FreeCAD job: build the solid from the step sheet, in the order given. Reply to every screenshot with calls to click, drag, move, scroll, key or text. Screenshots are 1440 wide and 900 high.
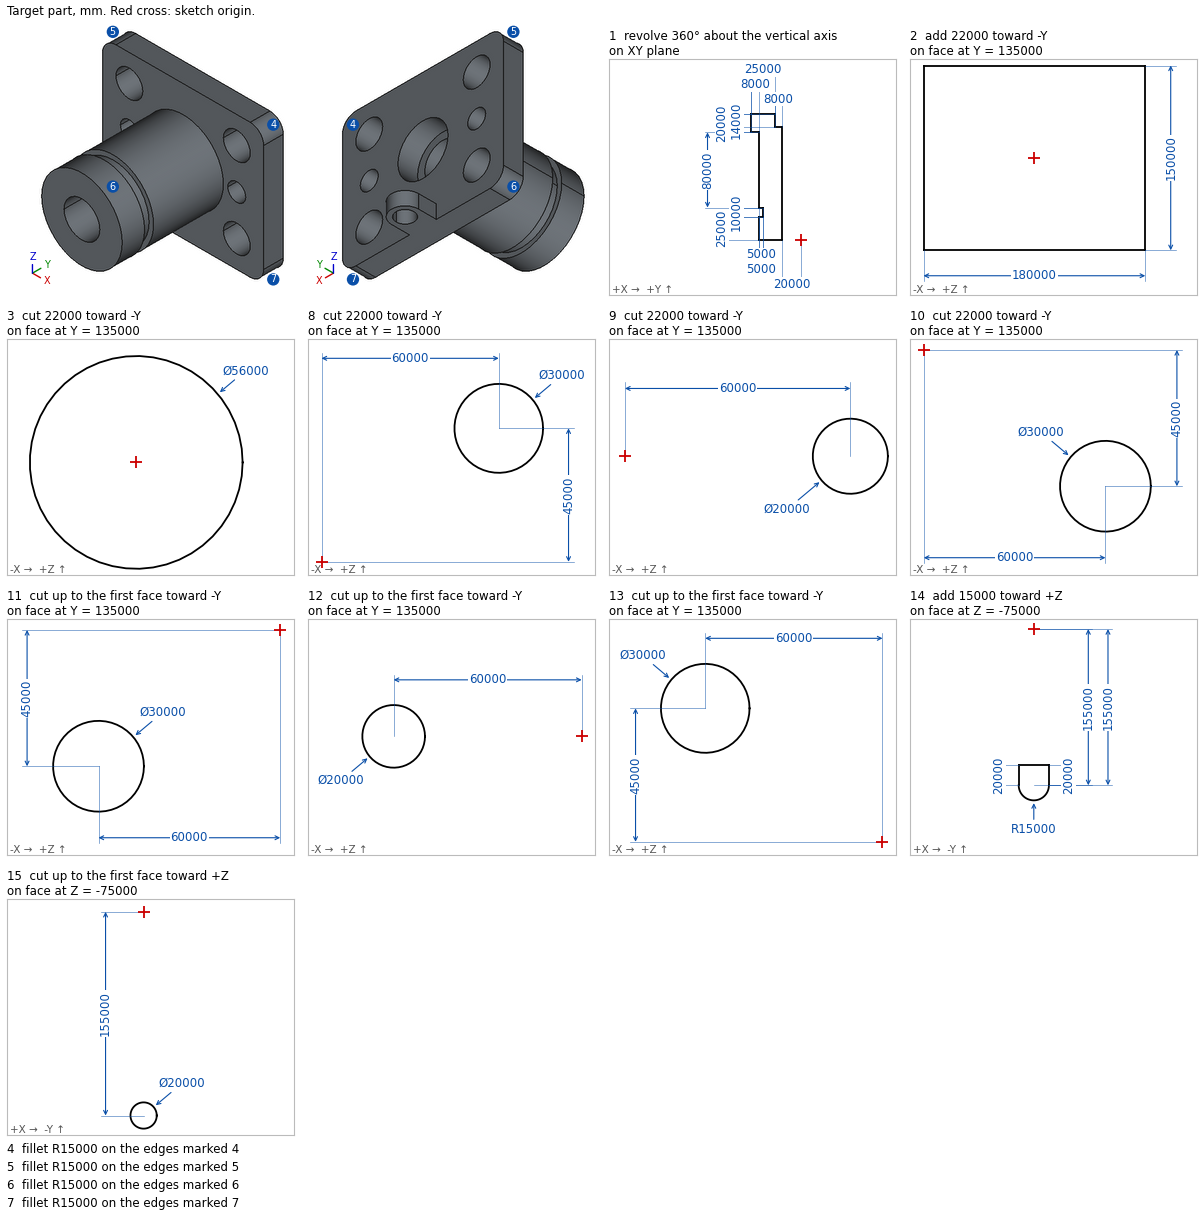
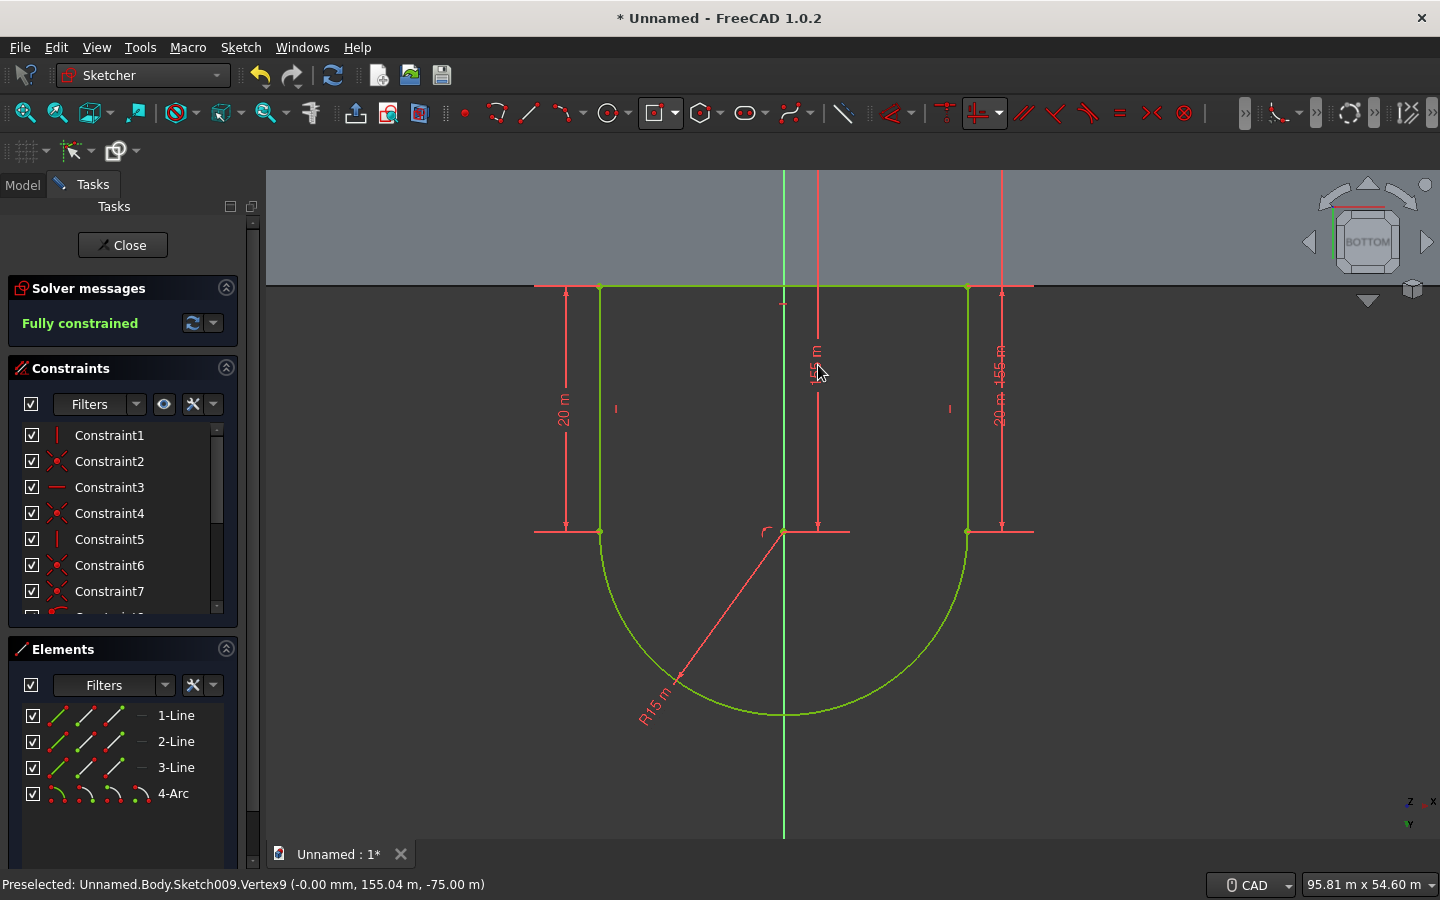
click(123, 245)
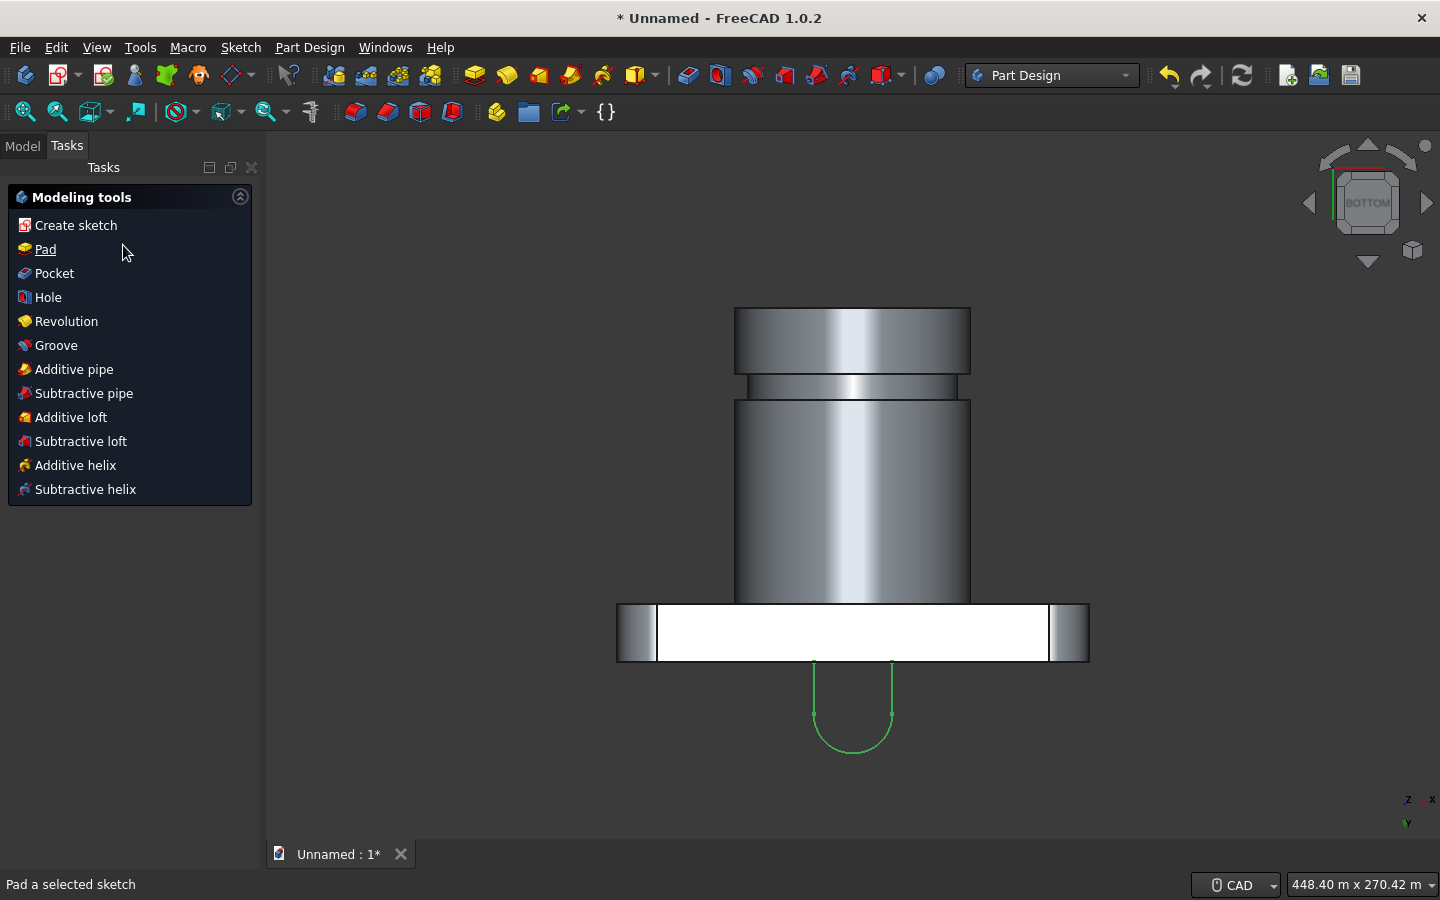
click(476, 76)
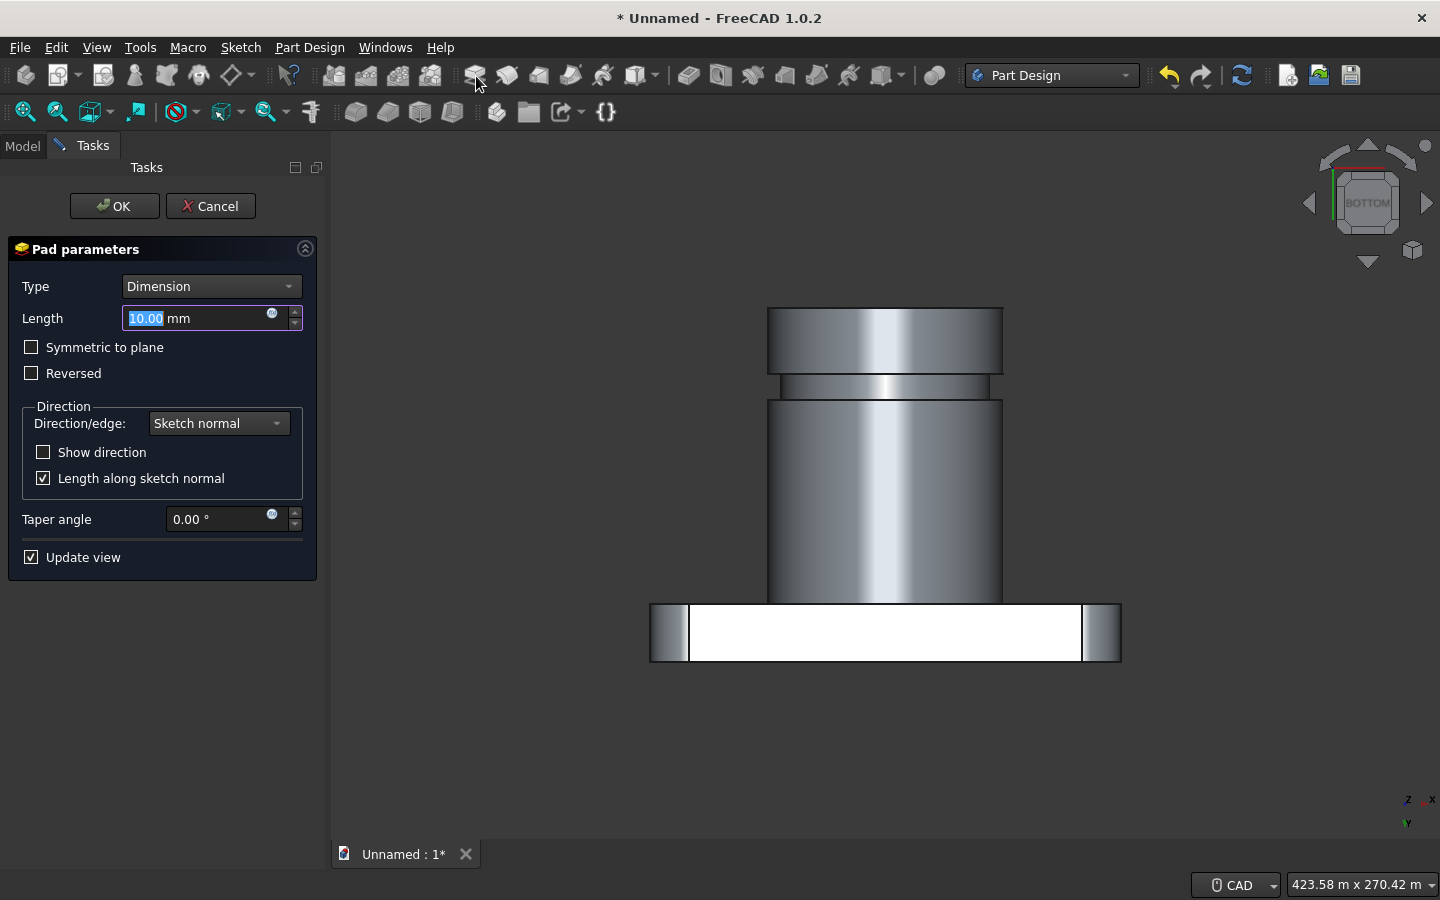
text(15000)
key(Tab)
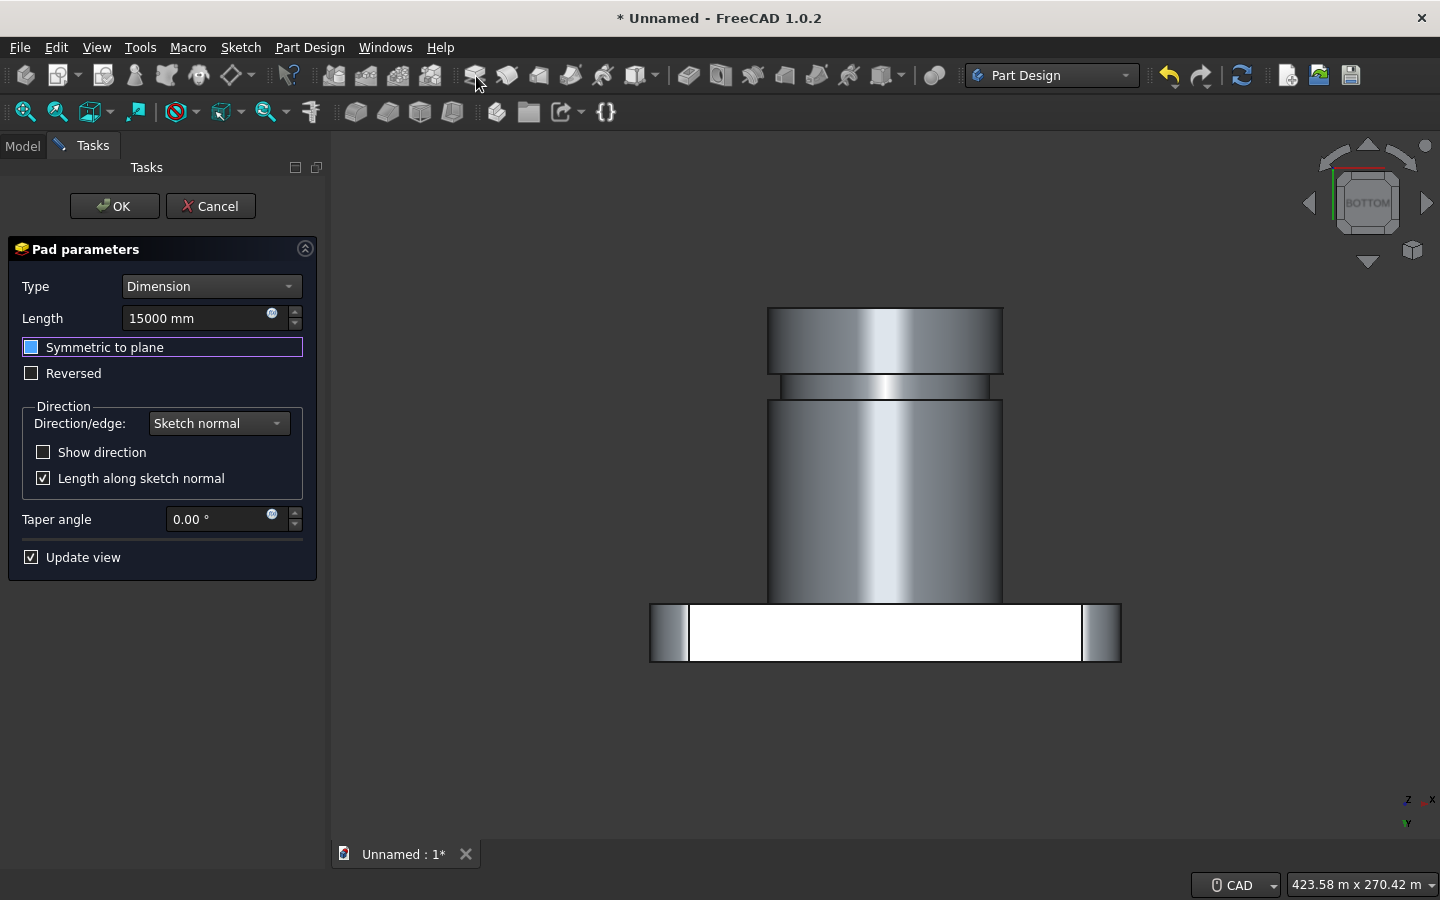
click(30, 373)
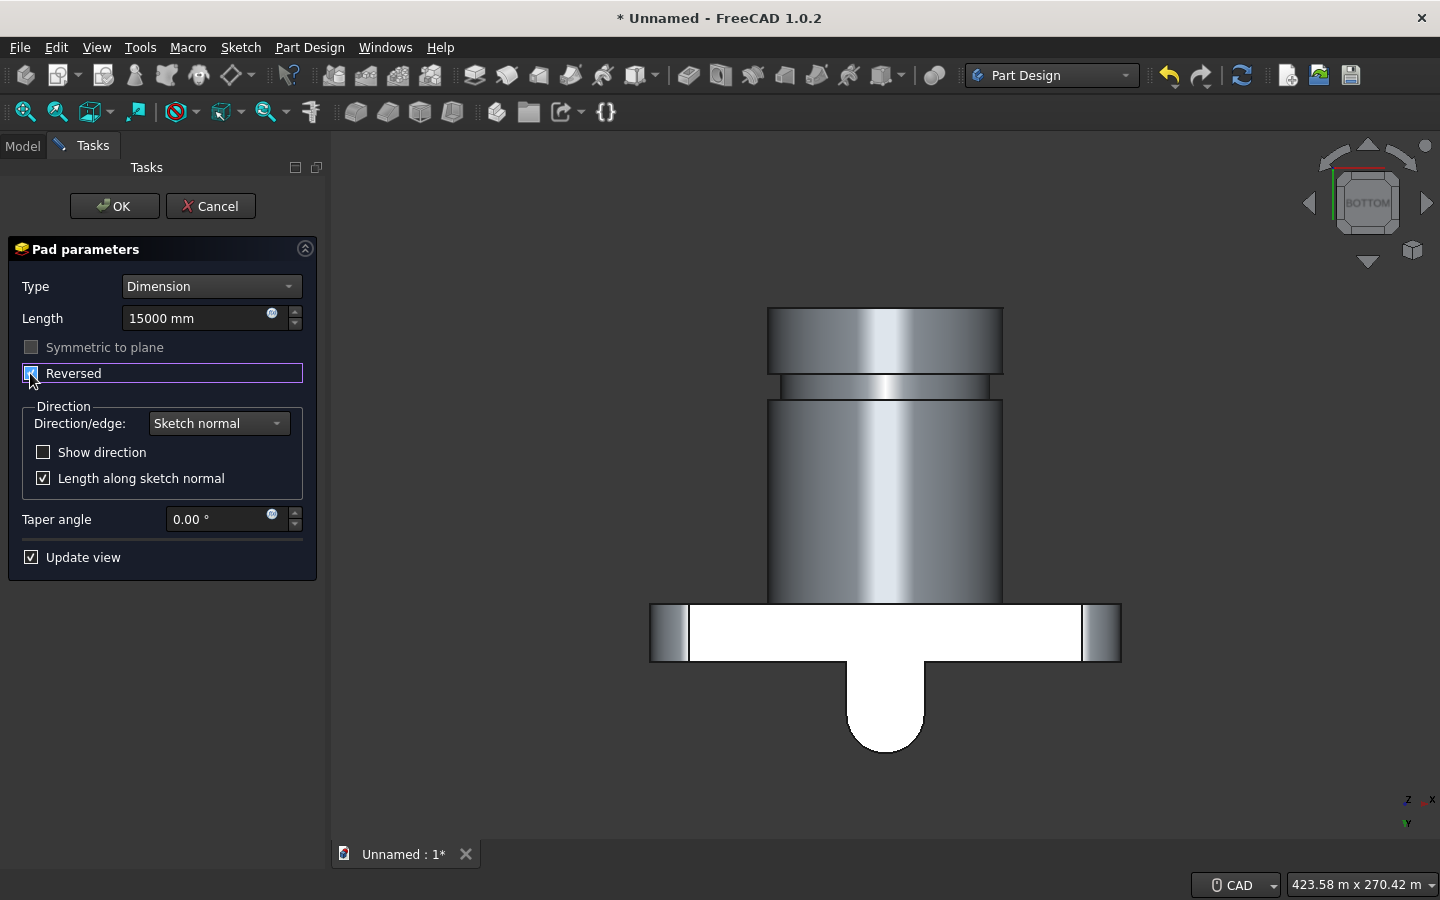
click(115, 206)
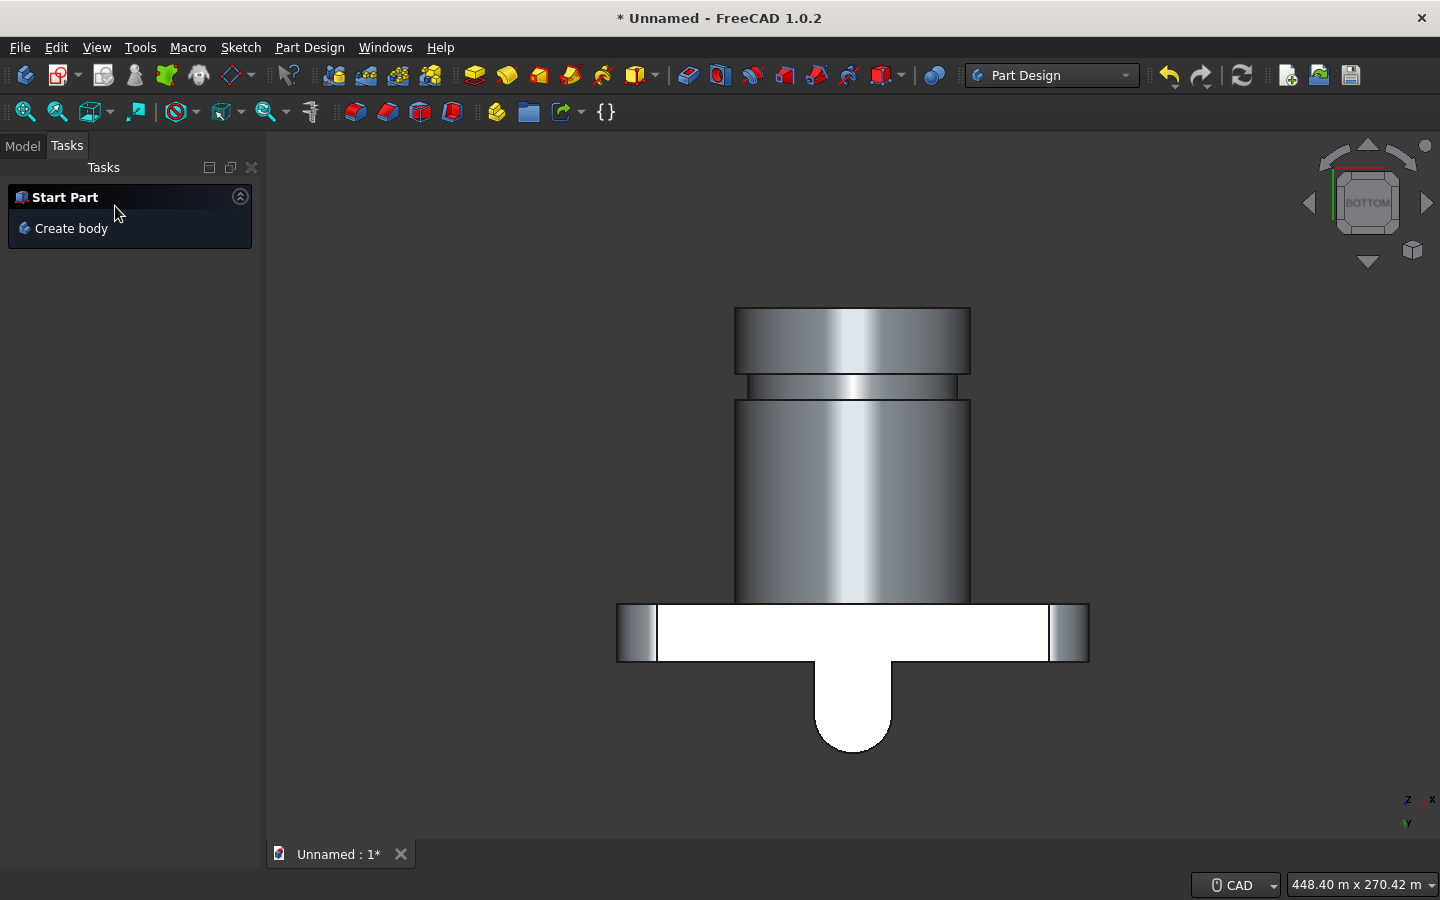
click(853, 656)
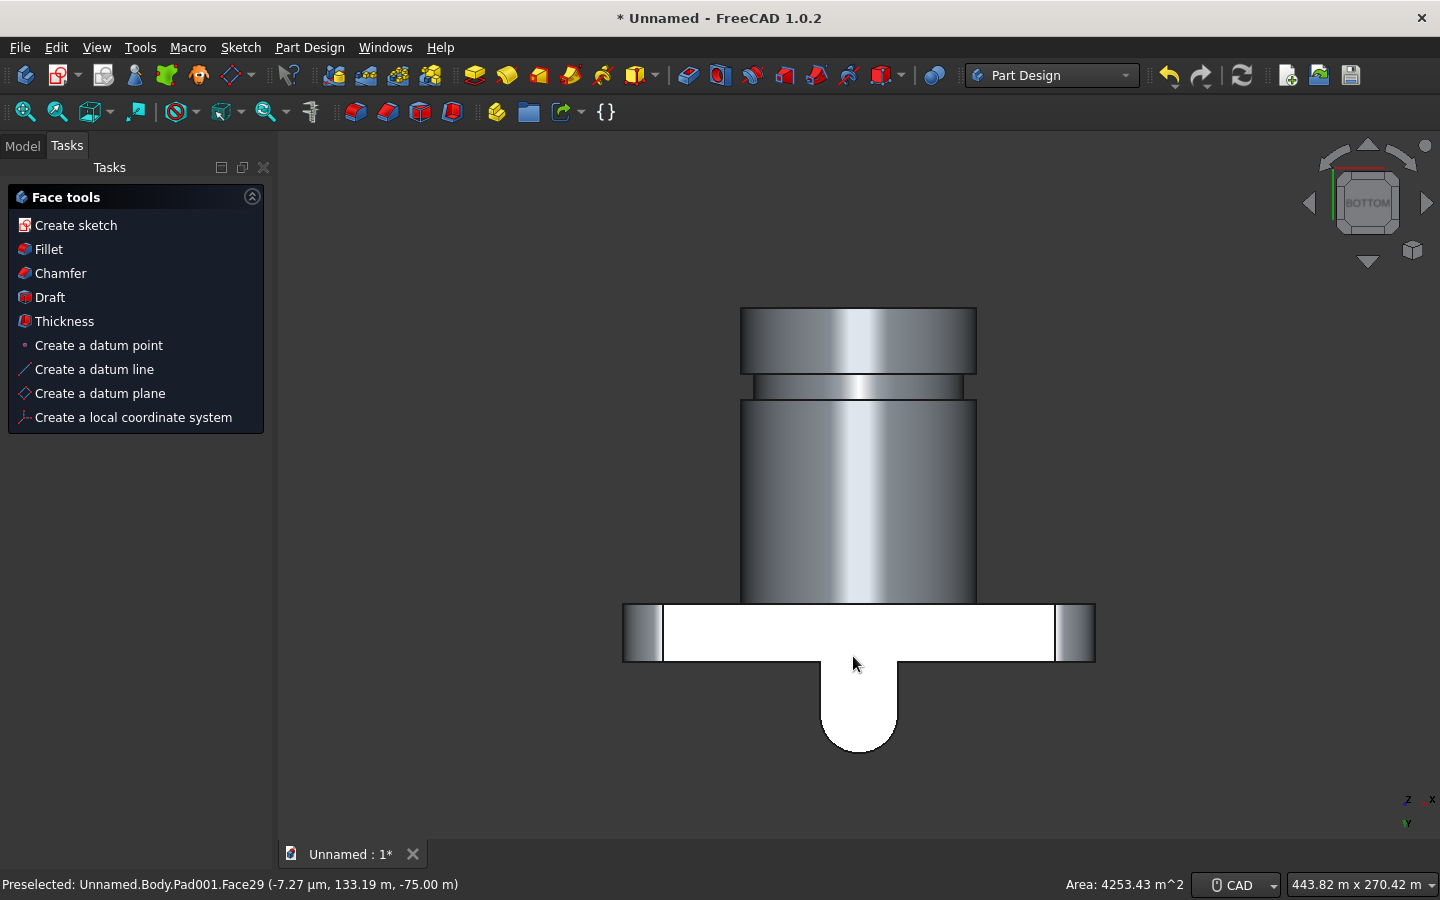
click(58, 76)